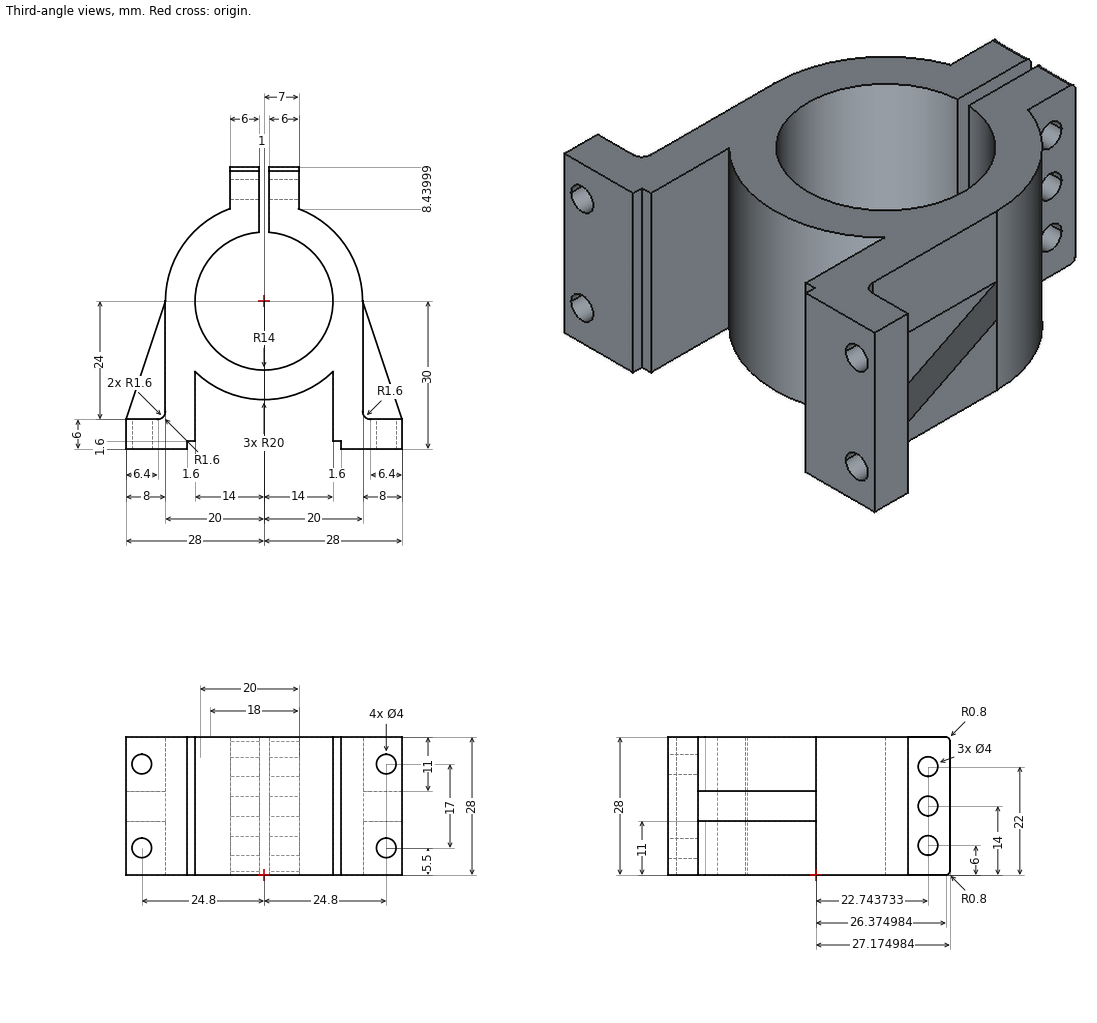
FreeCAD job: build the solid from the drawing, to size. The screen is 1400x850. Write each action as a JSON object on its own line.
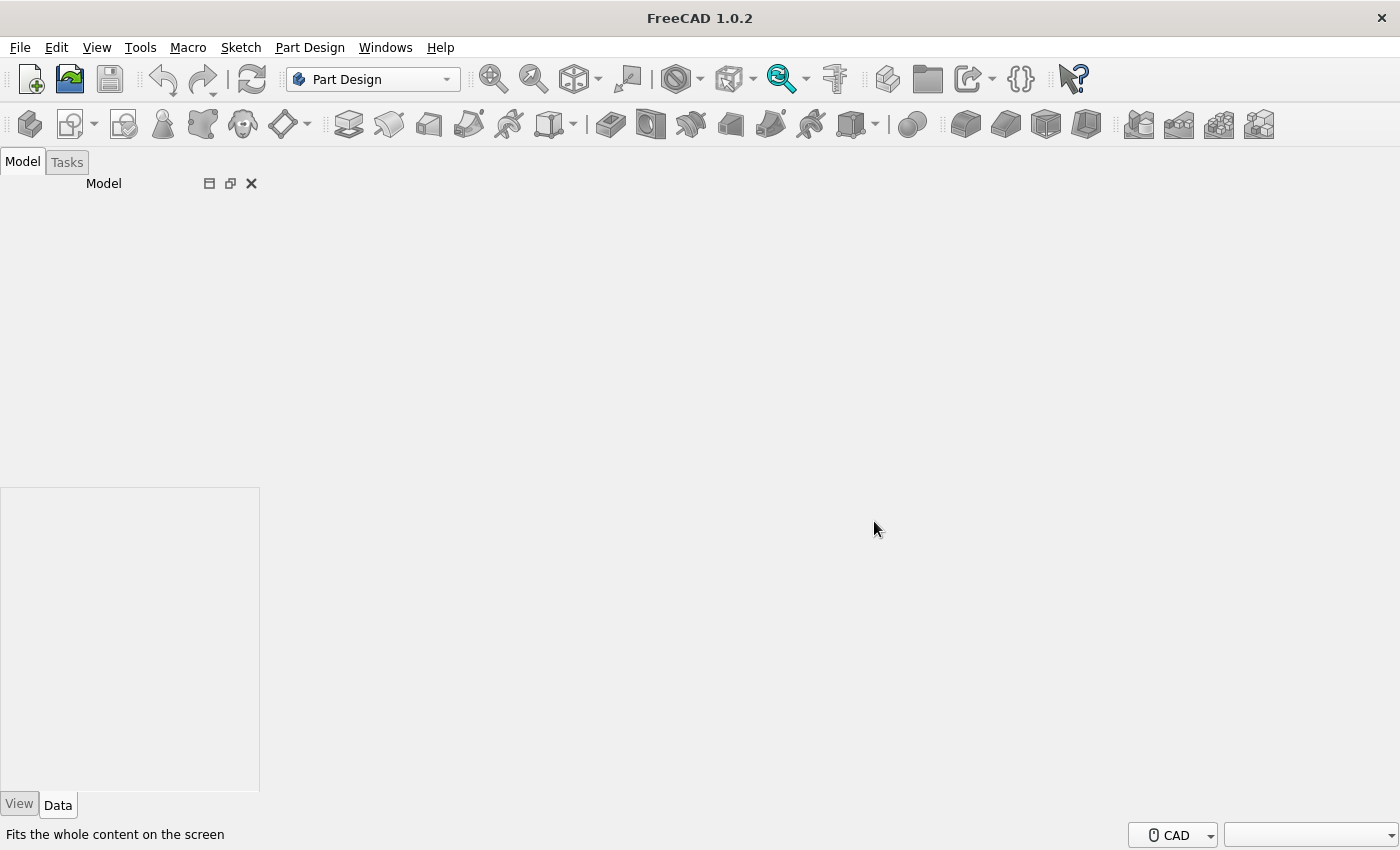
{"action": "left_click", "coordinate": [30, 80]}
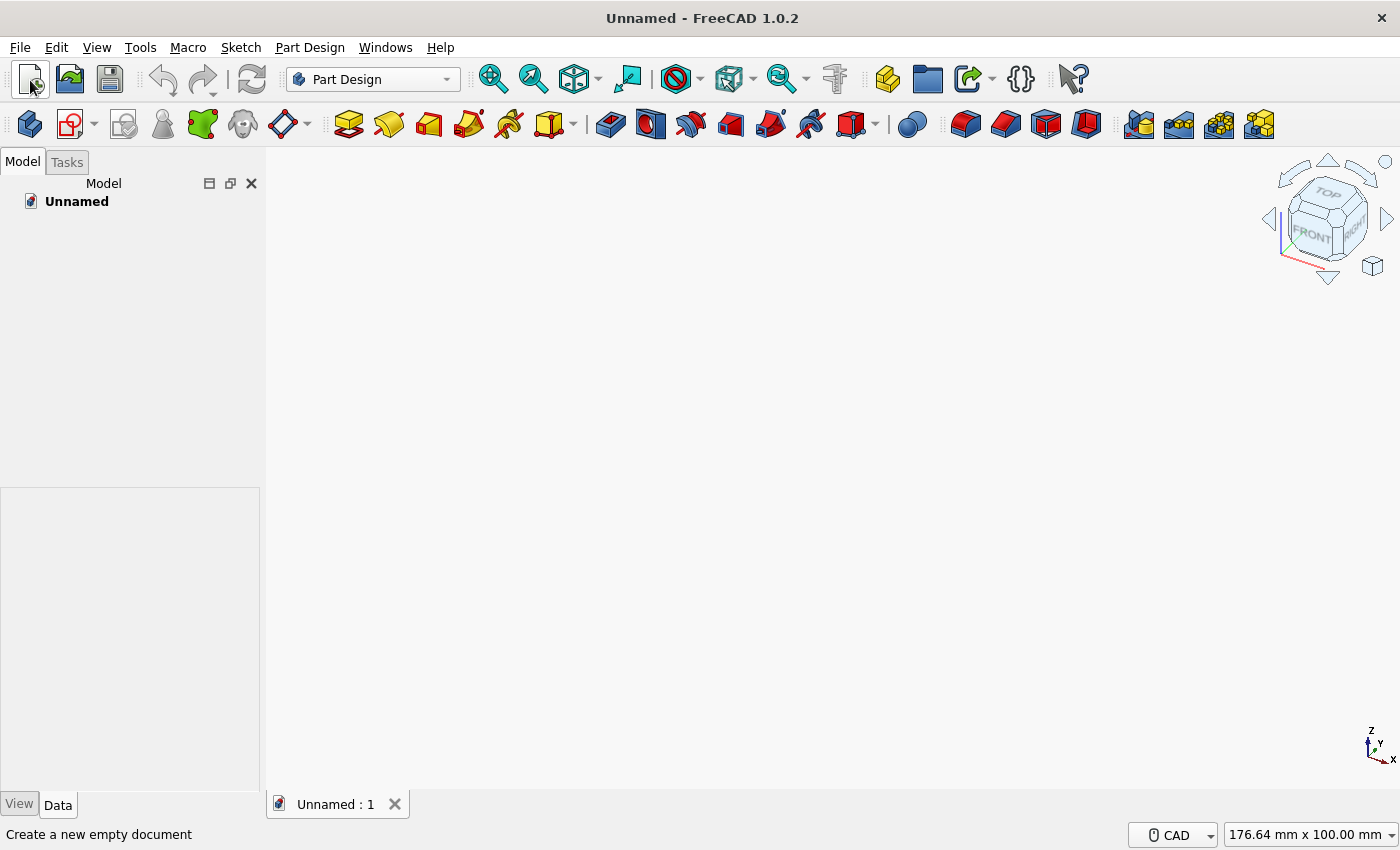
{"action": "left_click", "coordinate": [70, 124]}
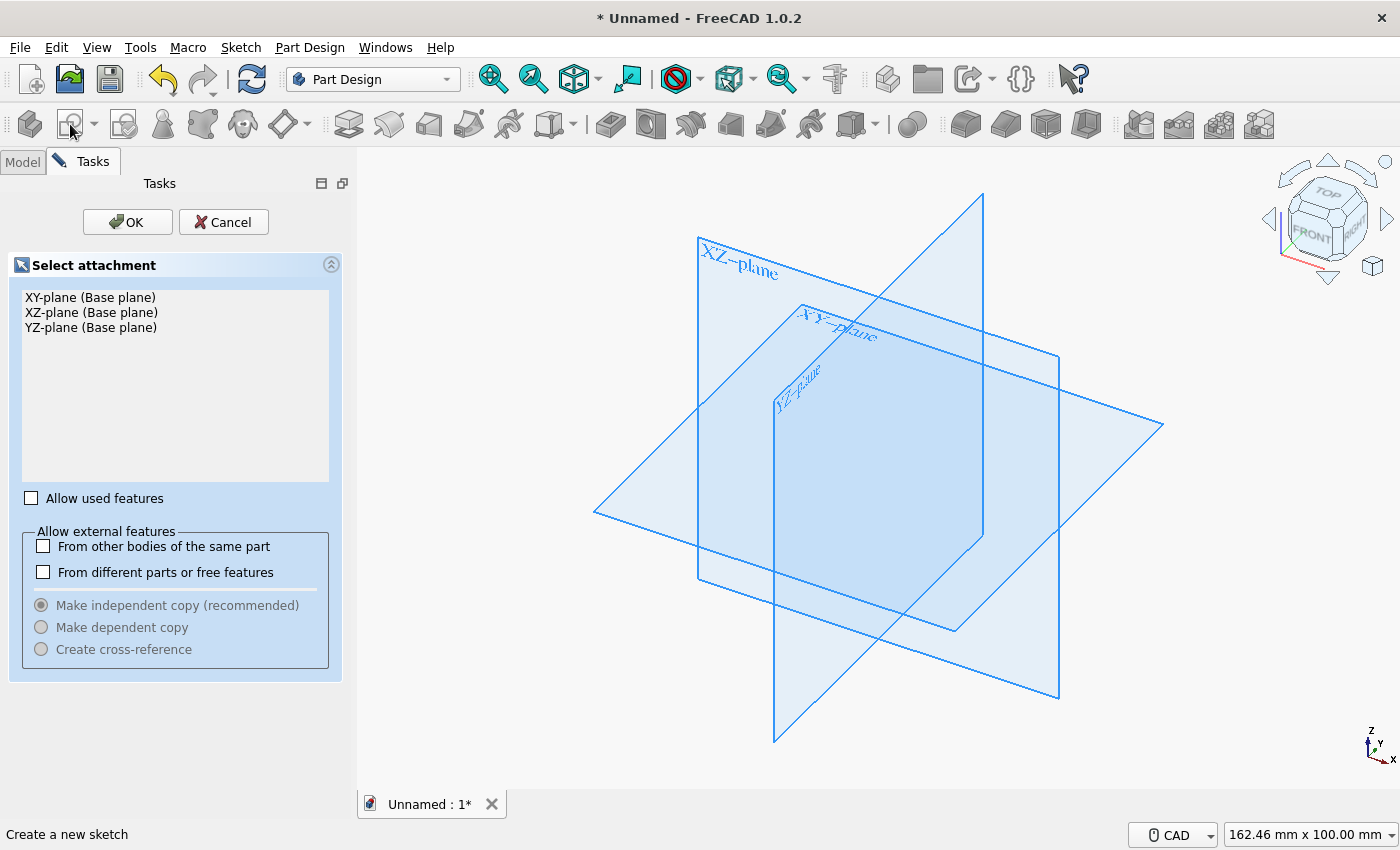
{"action": "left_click", "coordinate": [82, 298]}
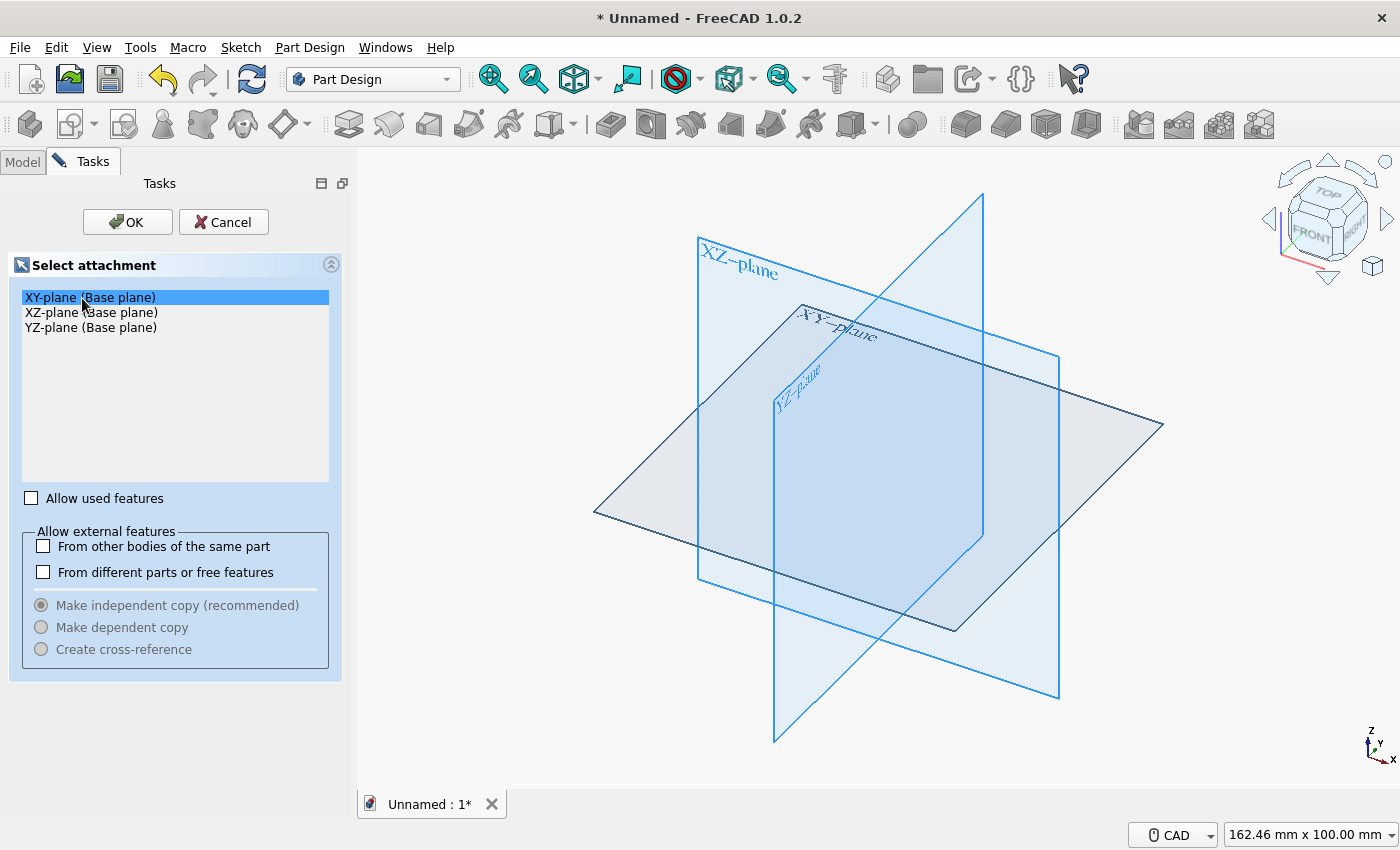
{"action": "left_click", "coordinate": [128, 222]}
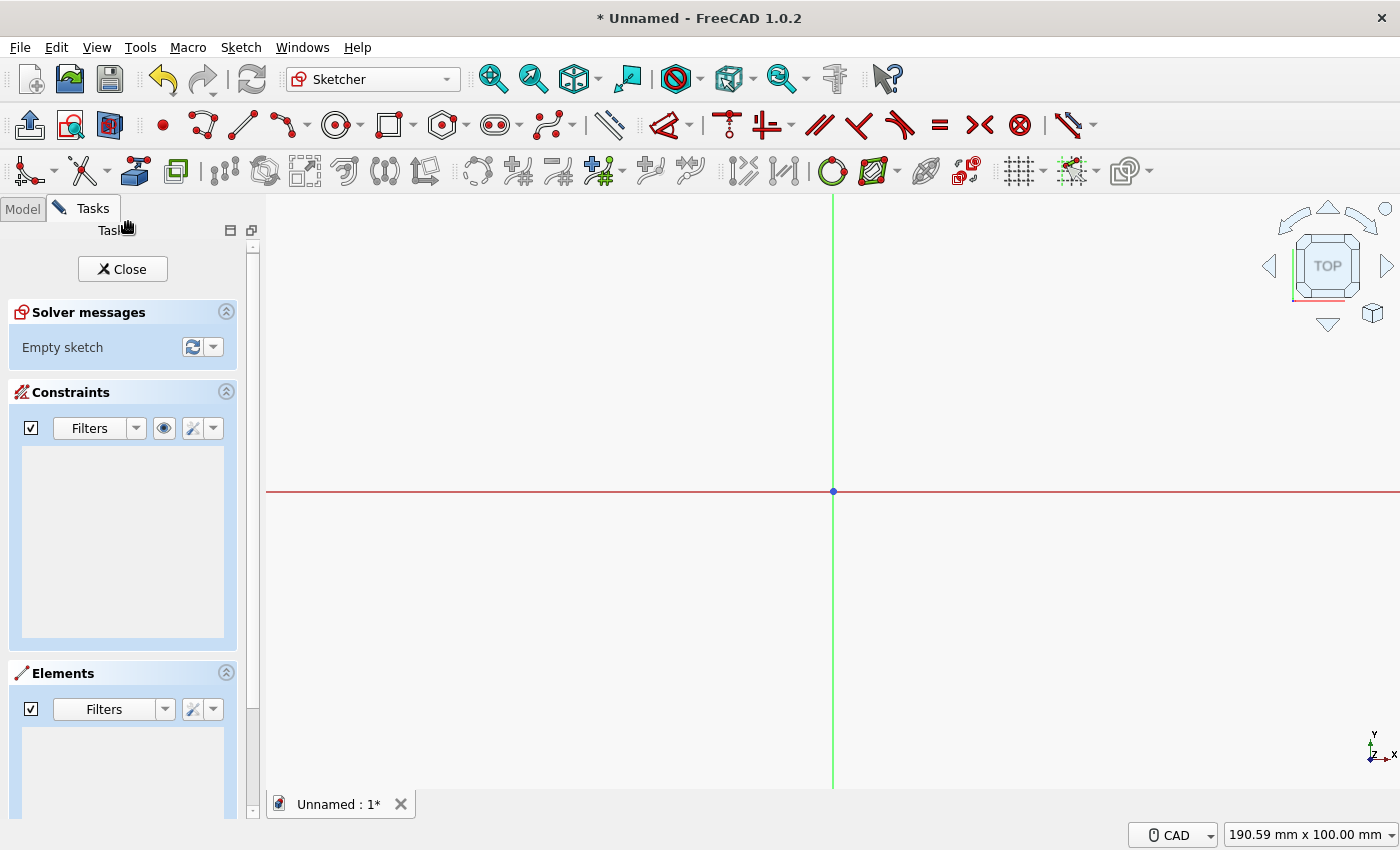
{"action": "left_click", "coordinate": [244, 126]}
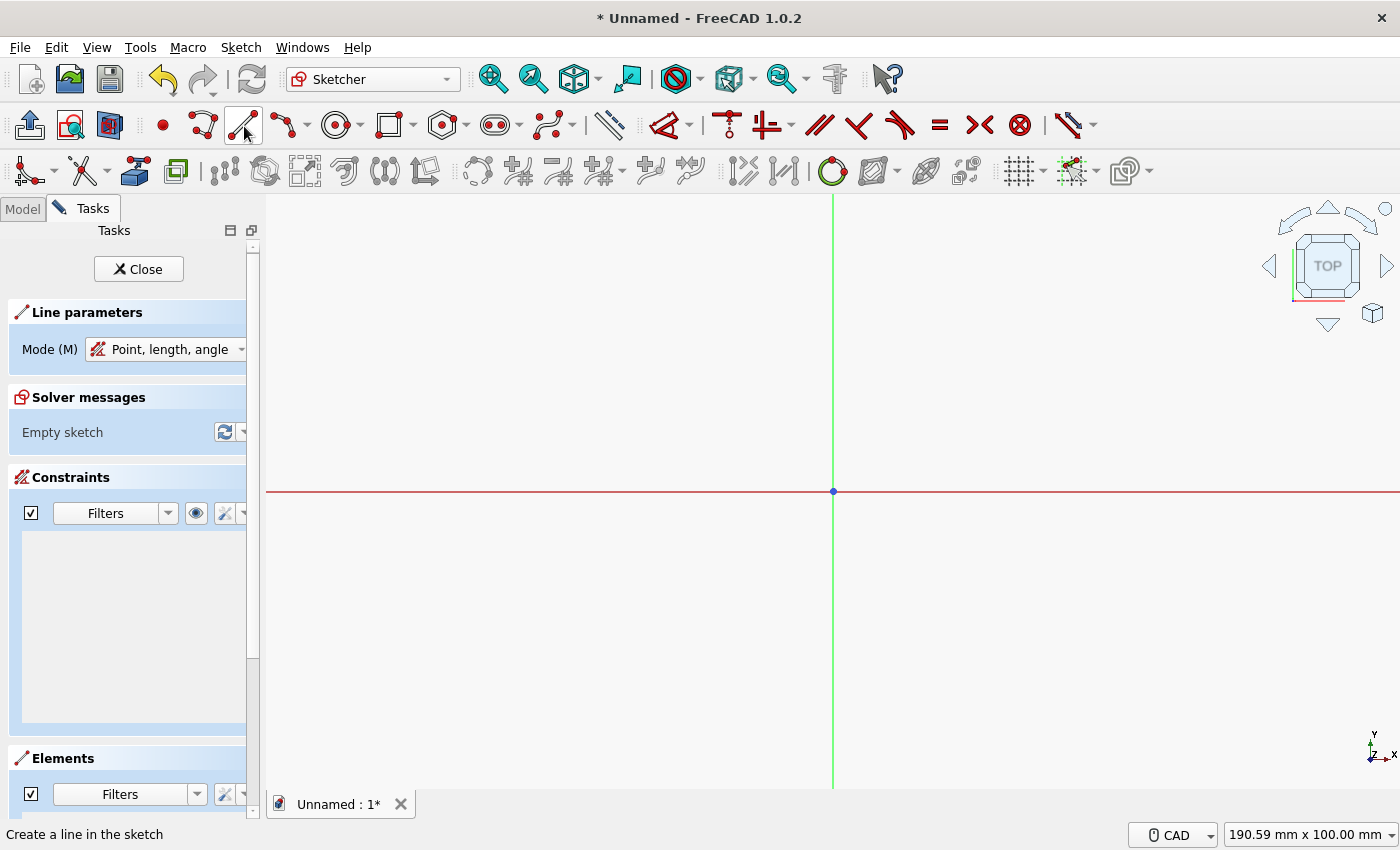
{"action": "left_click", "coordinate": [714, 492]}
{"action": "left_click", "coordinate": [714, 625]}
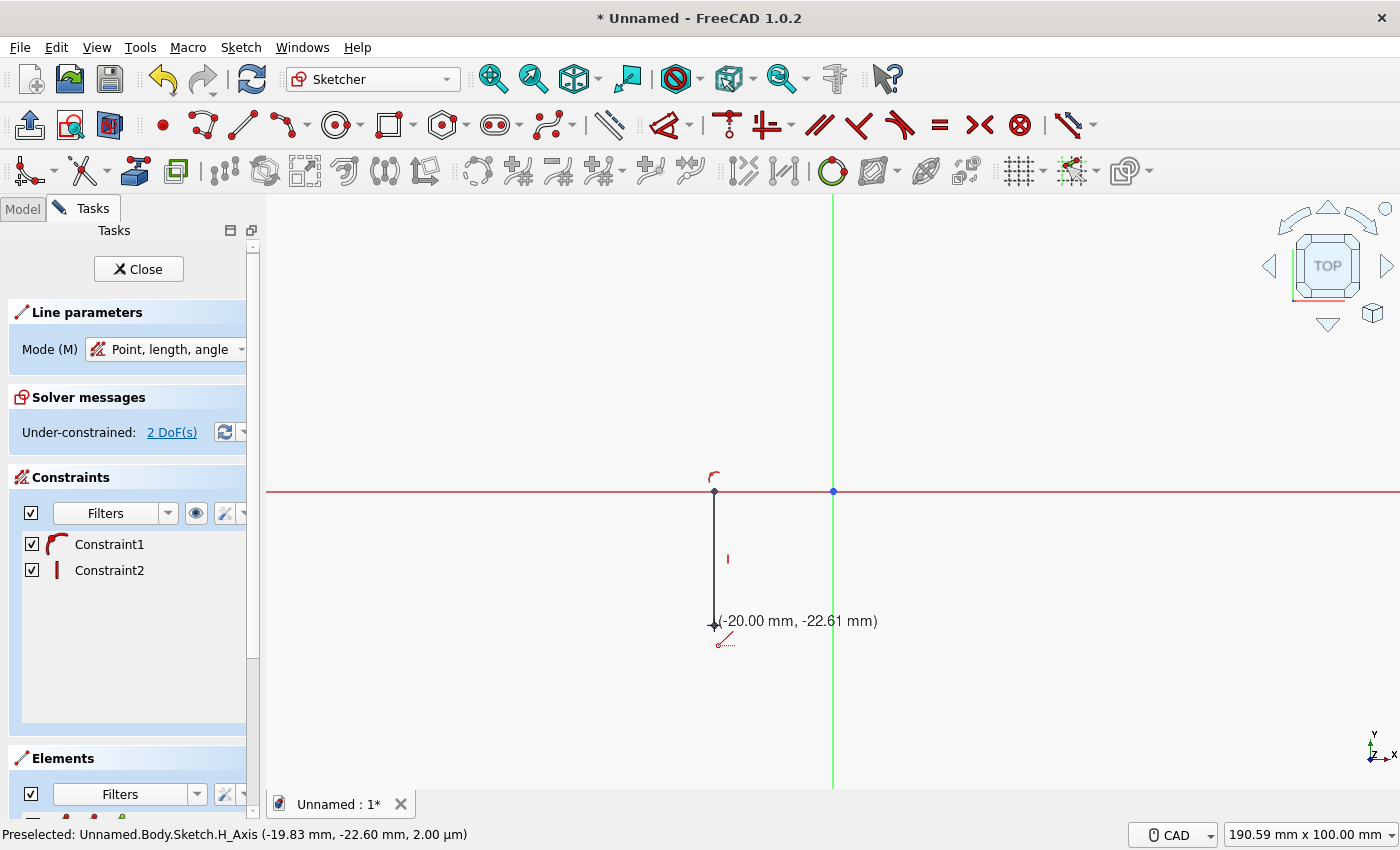
{"action": "left_click", "coordinate": [204, 126]}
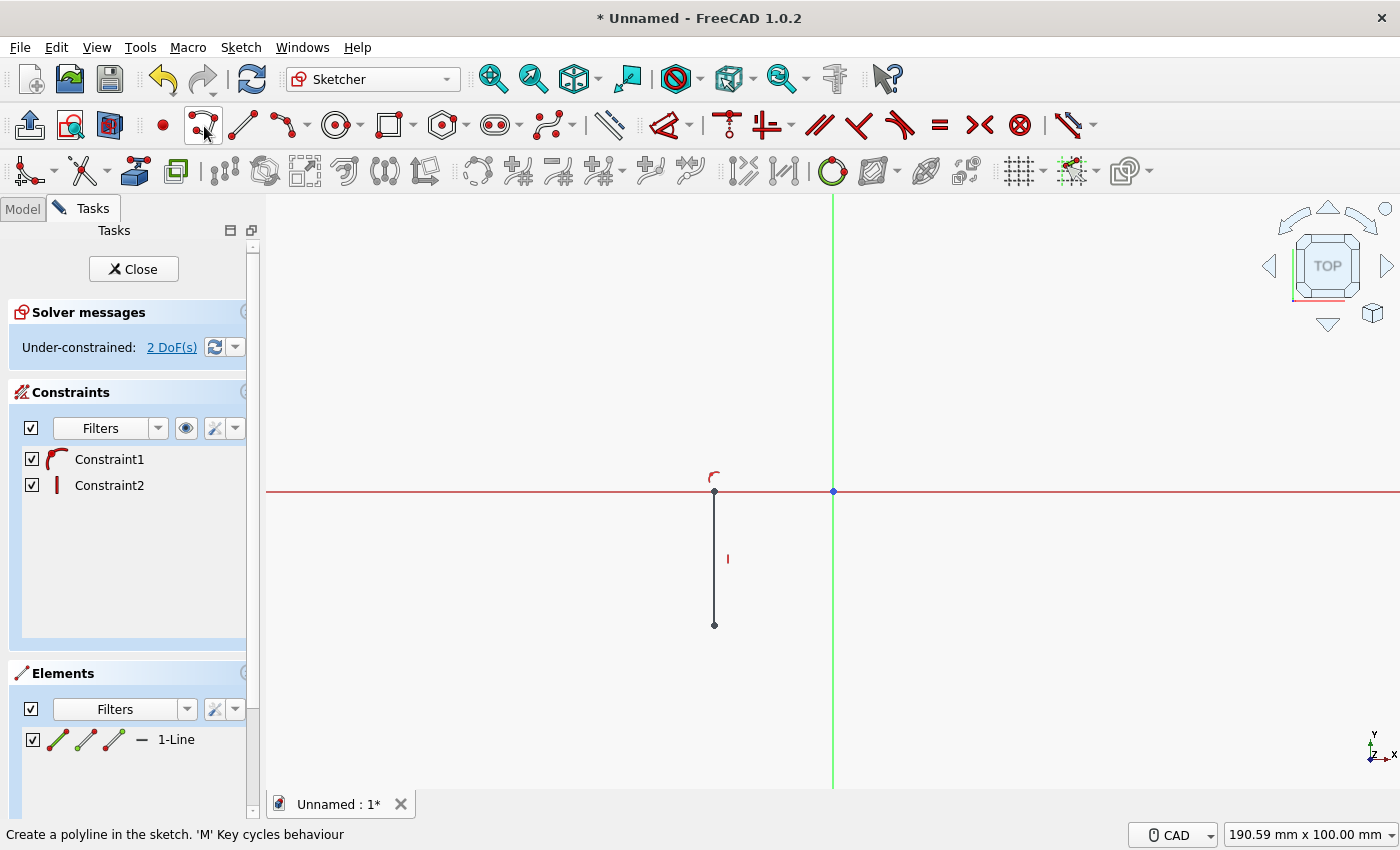
{"action": "left_click", "coordinate": [704, 634]}
{"action": "left_click", "coordinate": [666, 634]}
{"action": "left_click", "coordinate": [666, 670]}
{"action": "left_click", "coordinate": [740, 670]}